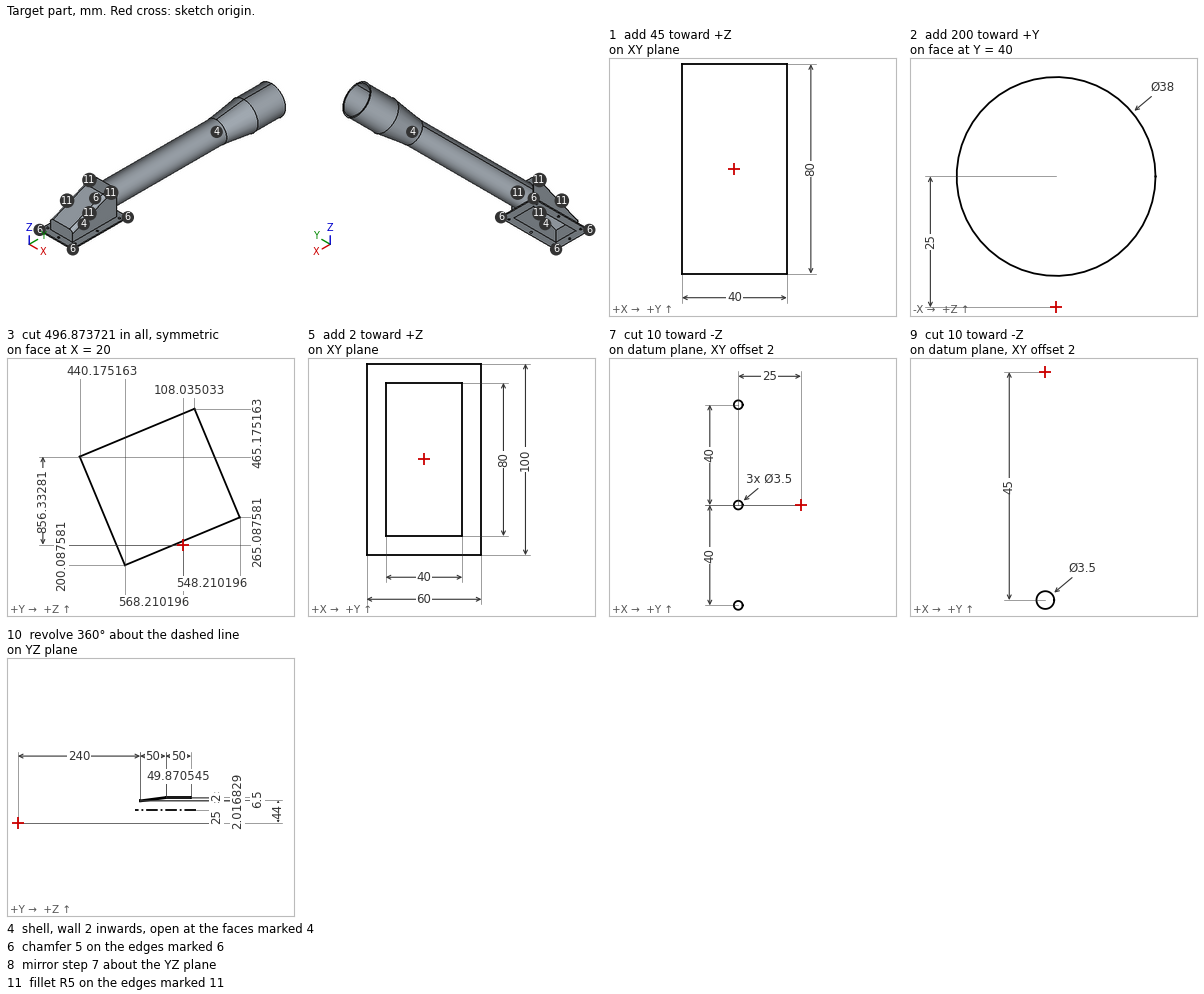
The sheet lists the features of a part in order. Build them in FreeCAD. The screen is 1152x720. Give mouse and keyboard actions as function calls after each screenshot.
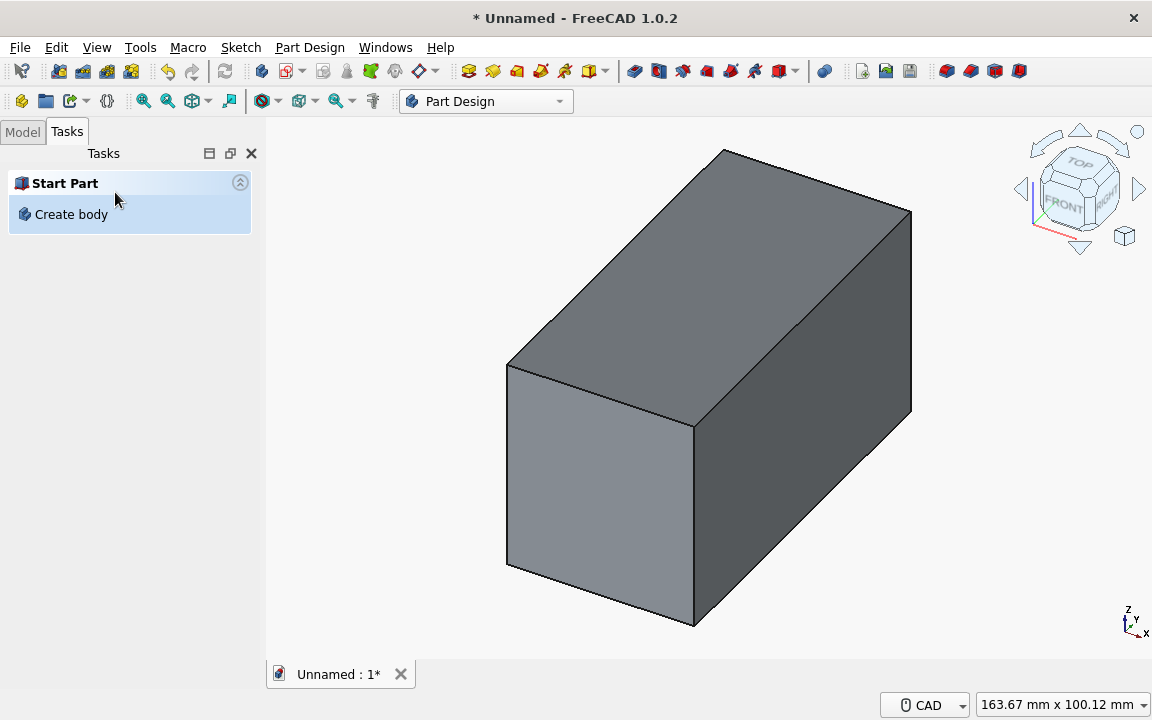
key(4)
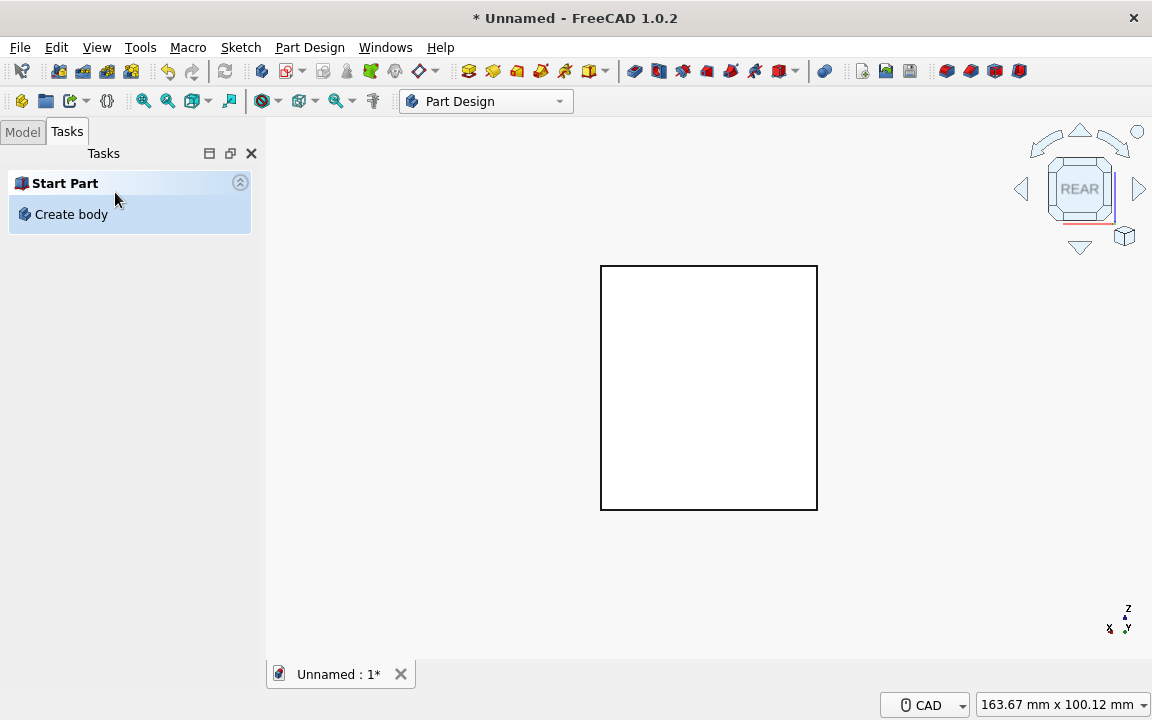
click(709, 387)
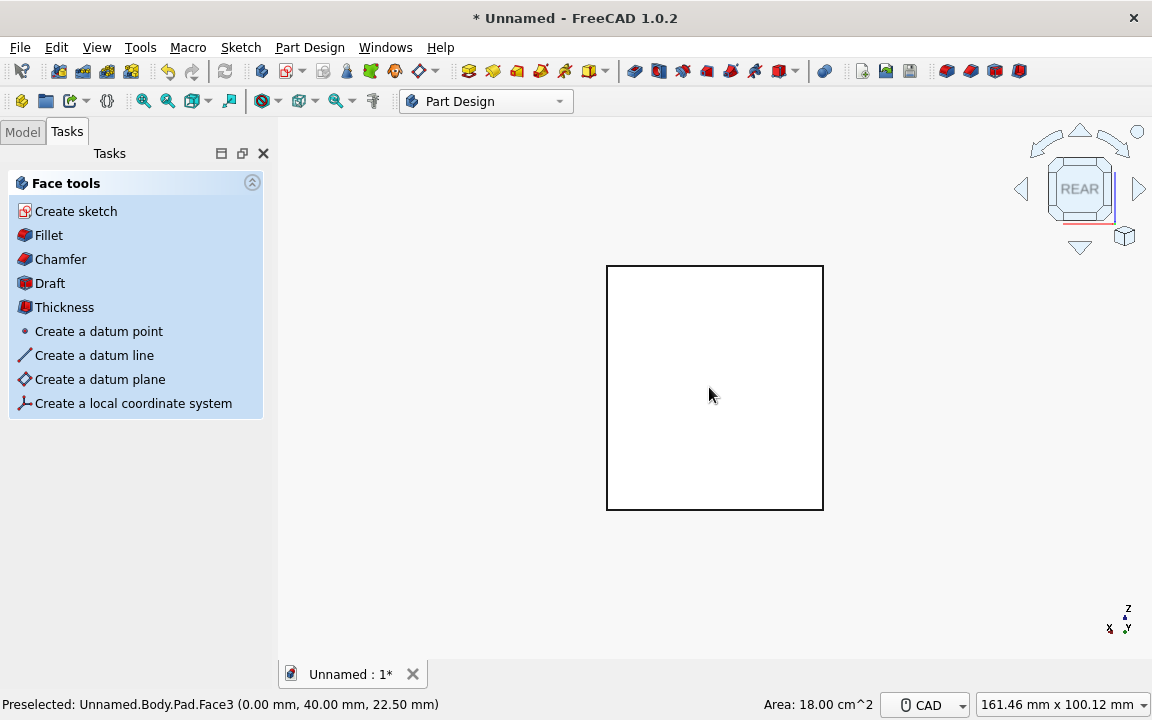
click(286, 72)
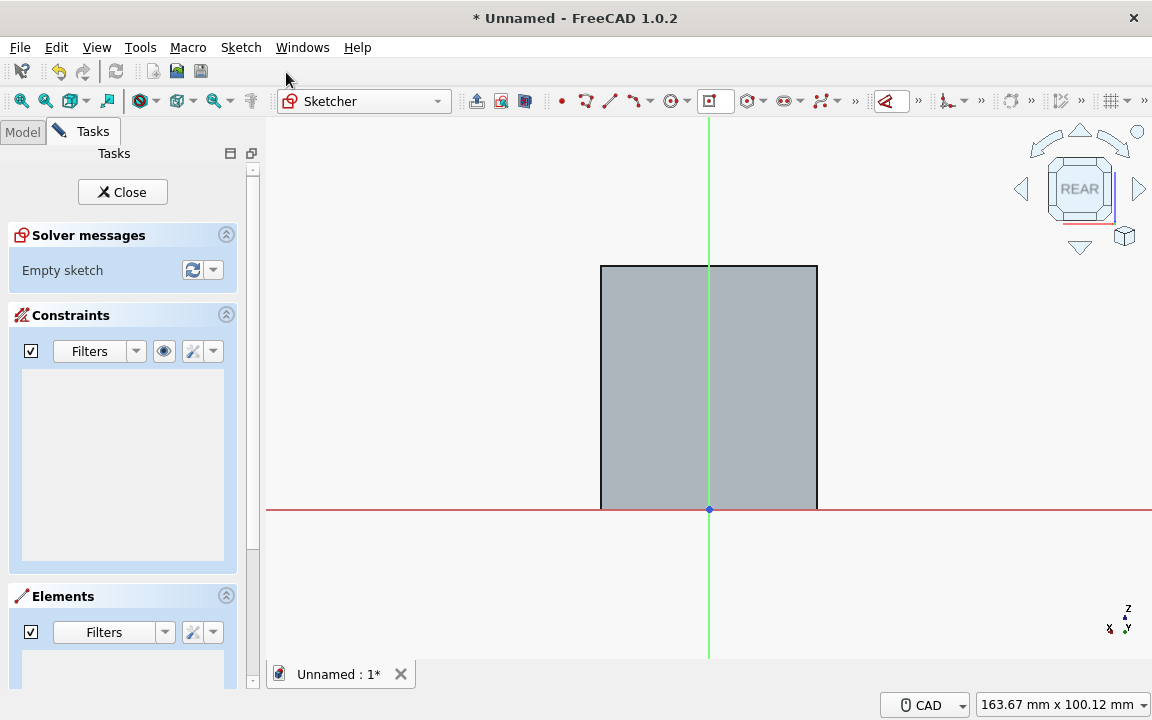
scroll(848, 396, up, 2)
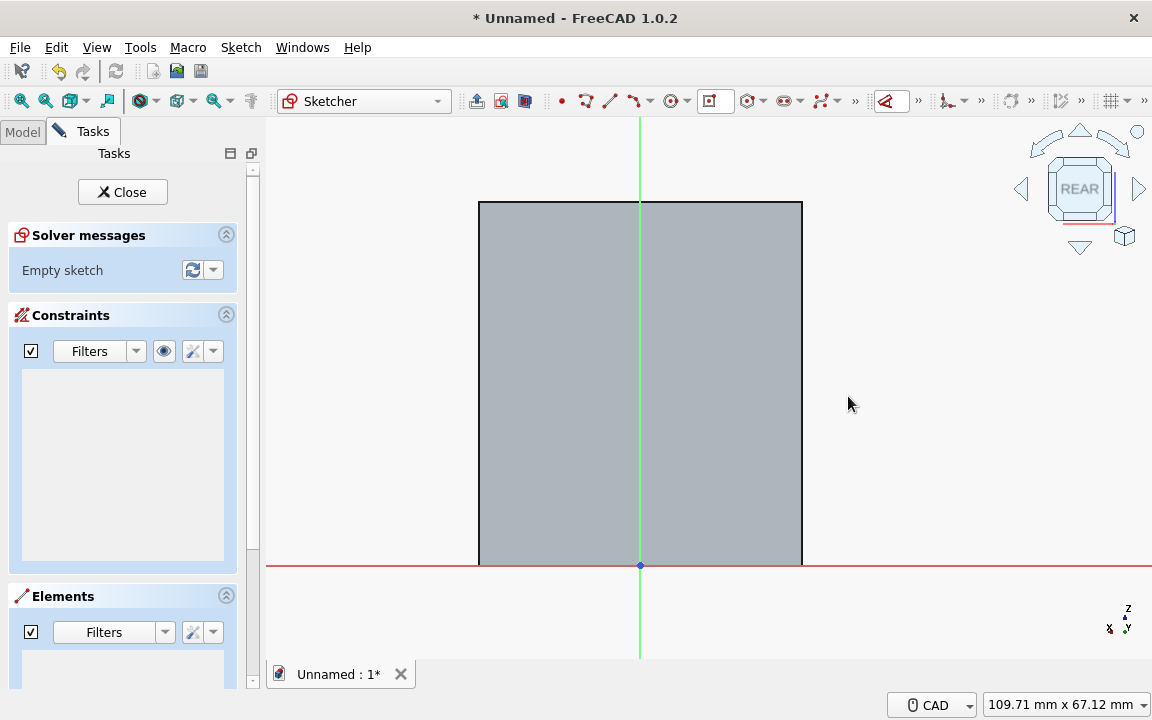
click(672, 102)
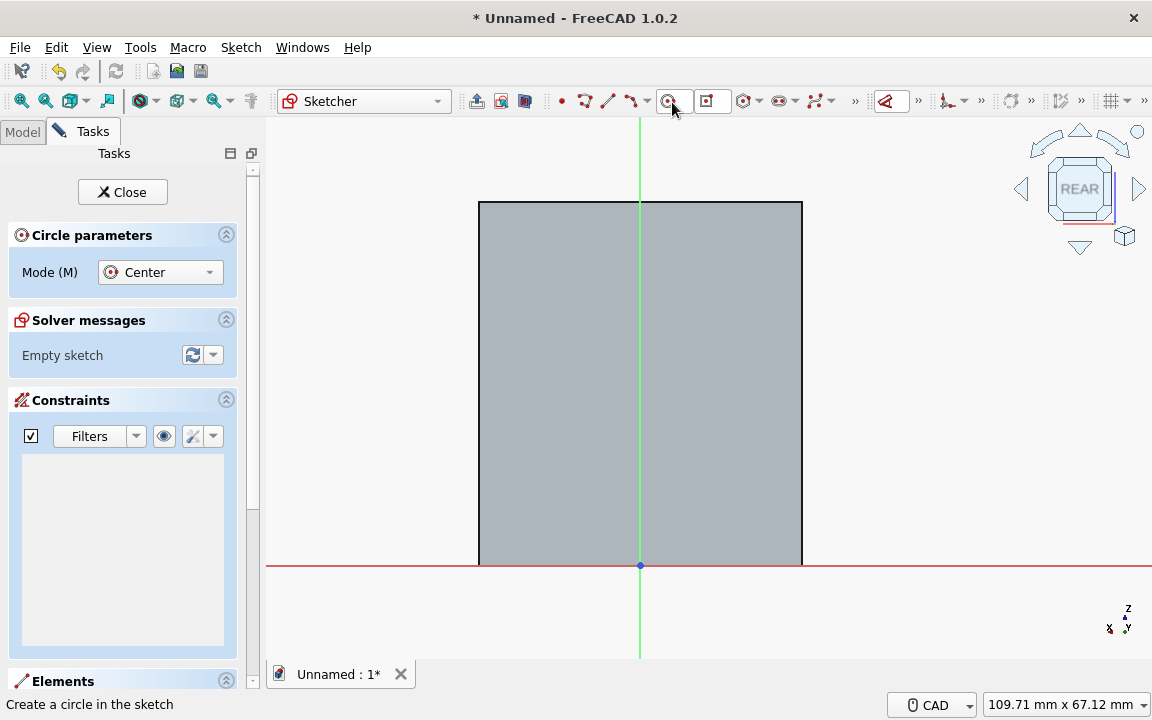
click(640, 364)
move(749, 255)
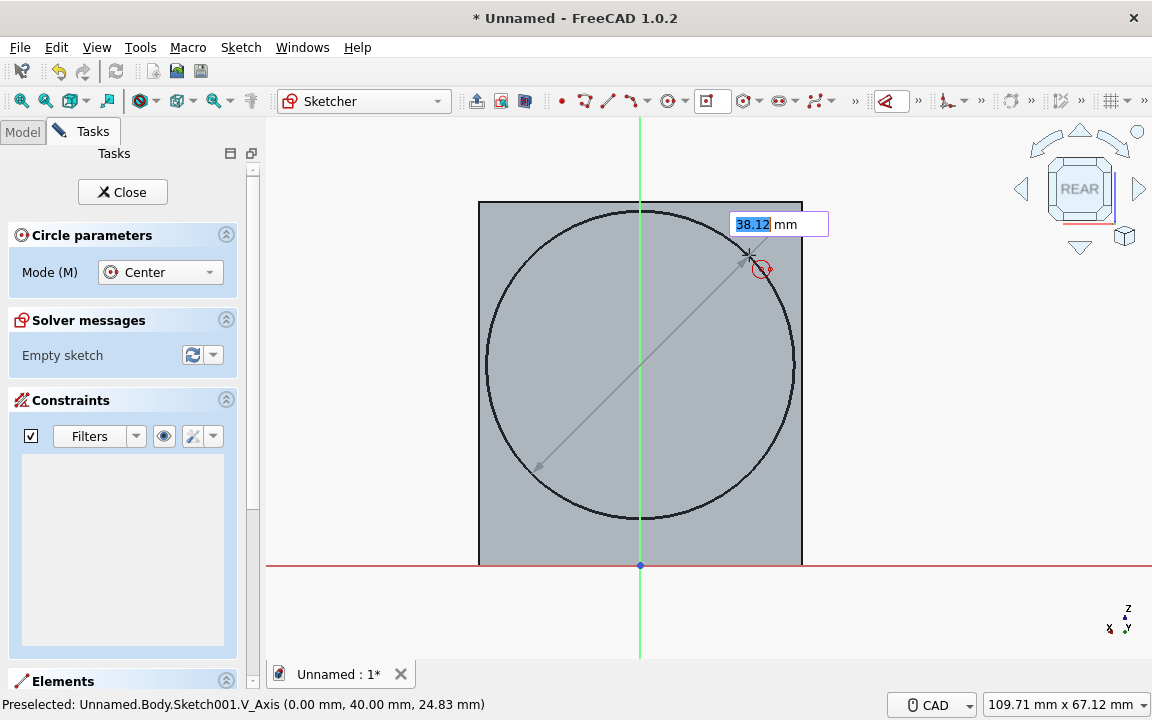
text(38)
key(Return)
key(Escape)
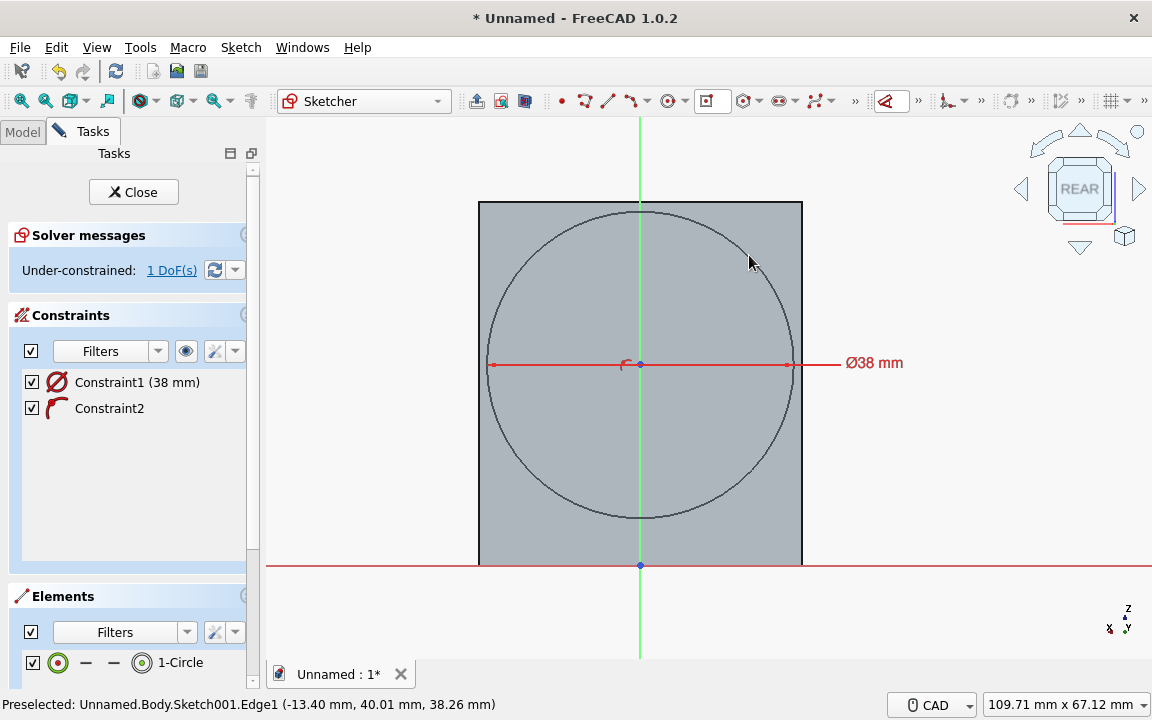
key(d)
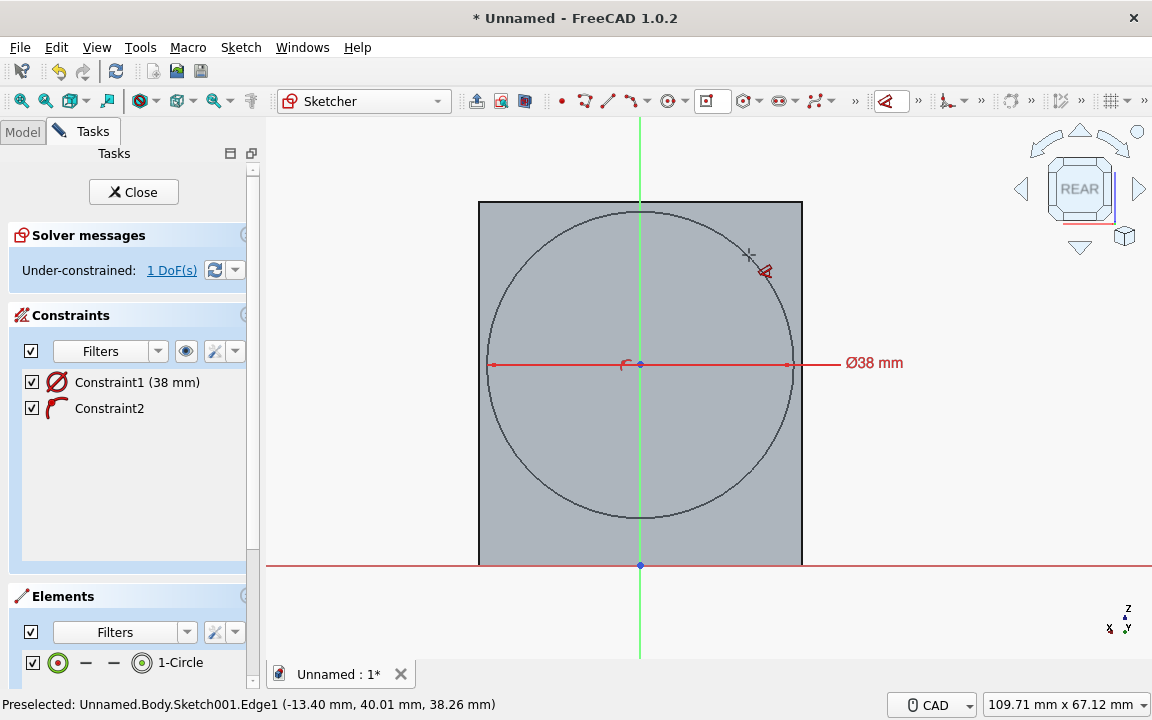
click(640, 365)
click(674, 465)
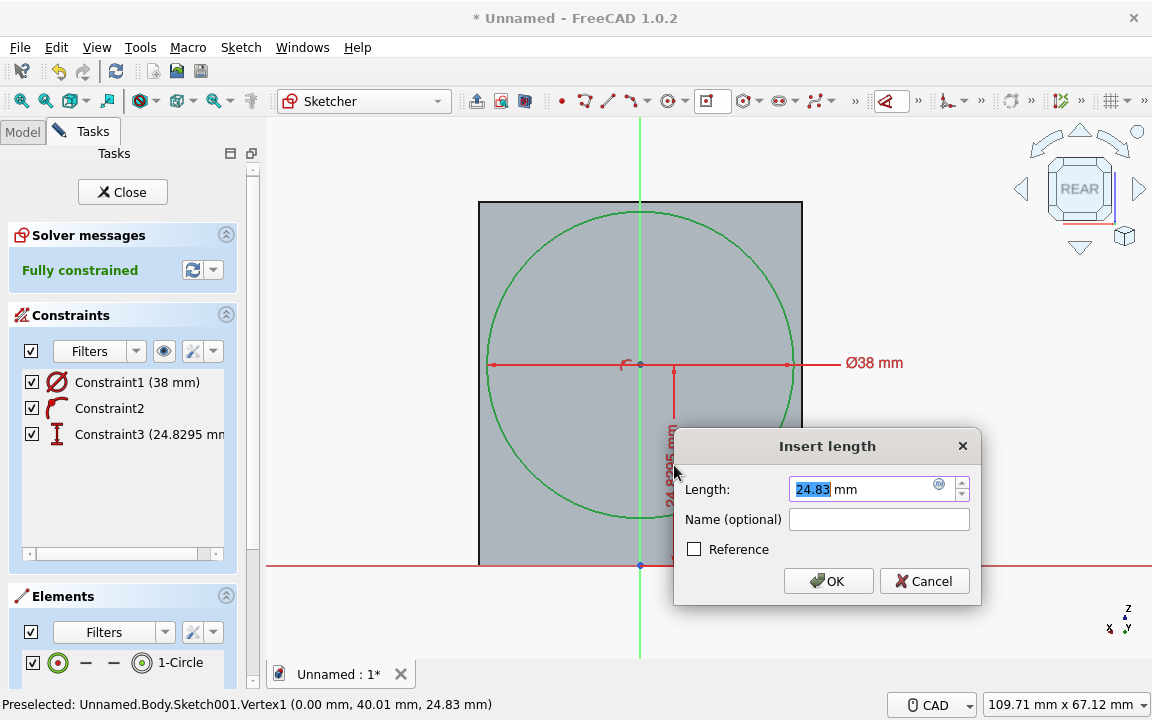
text(25)
key(Return)
key(Escape)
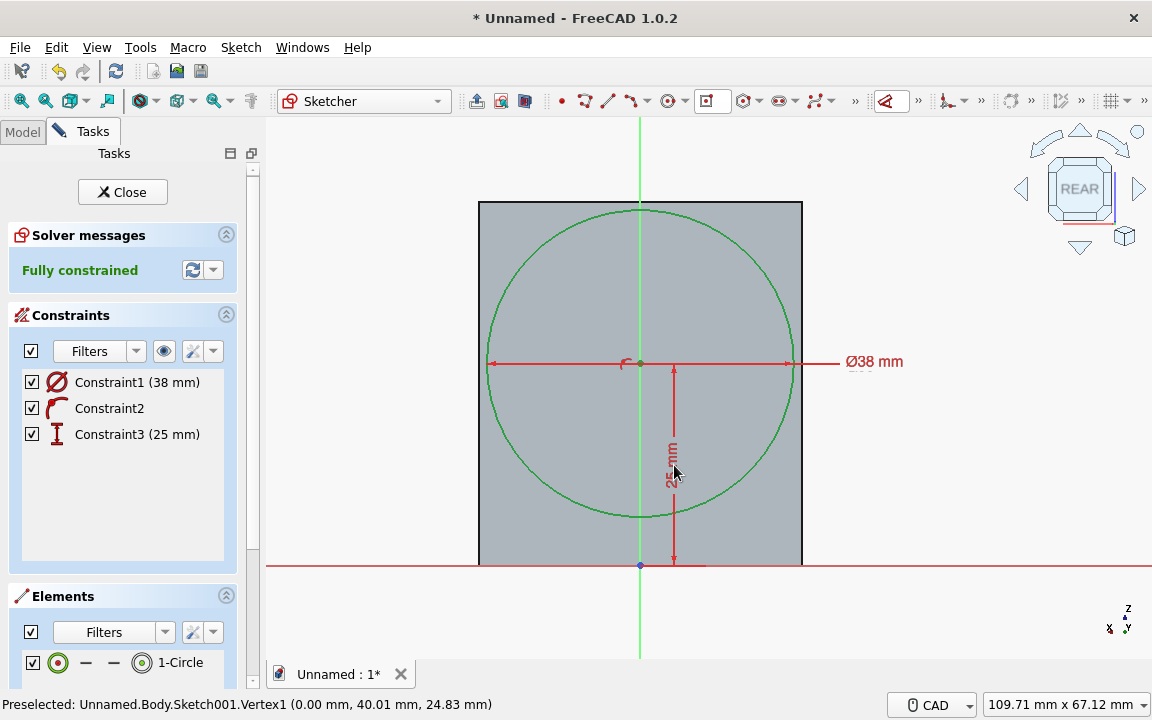
click(123, 192)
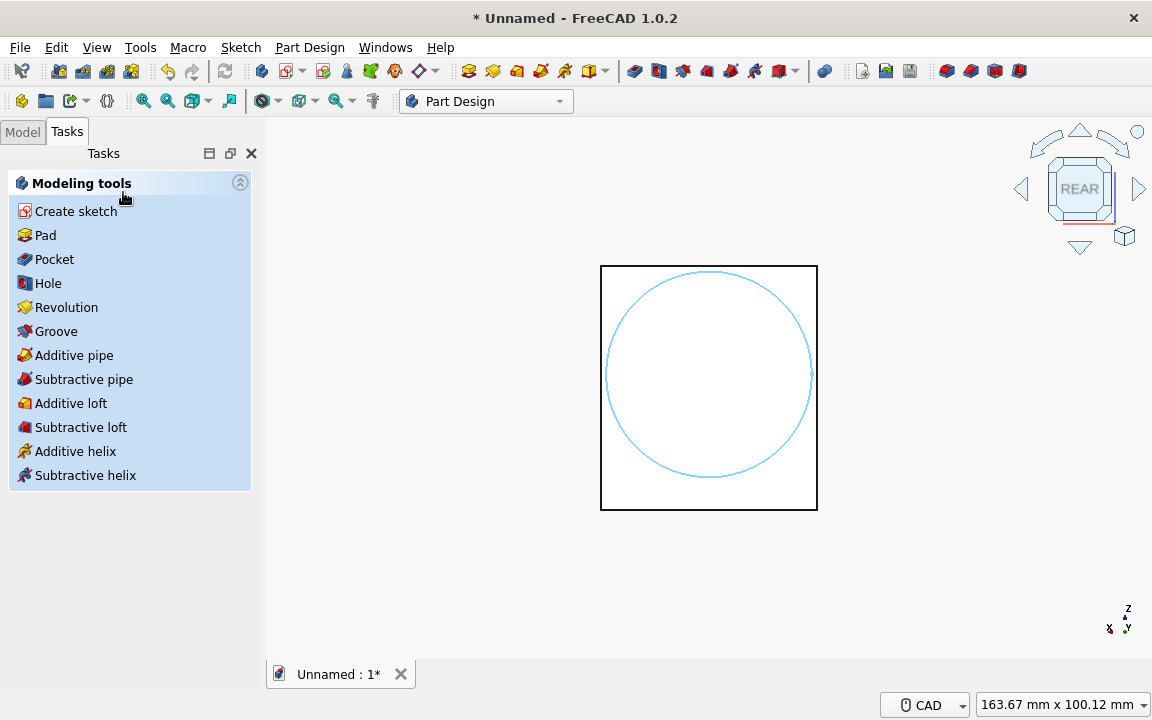
click(470, 72)